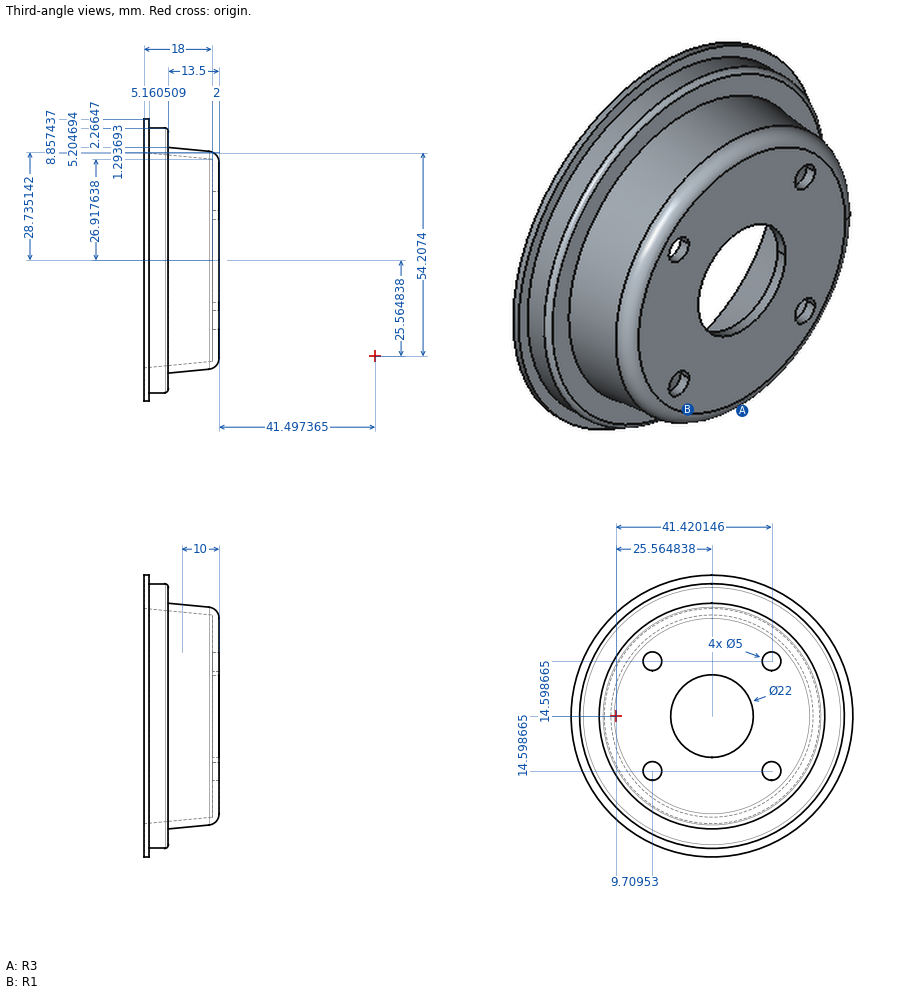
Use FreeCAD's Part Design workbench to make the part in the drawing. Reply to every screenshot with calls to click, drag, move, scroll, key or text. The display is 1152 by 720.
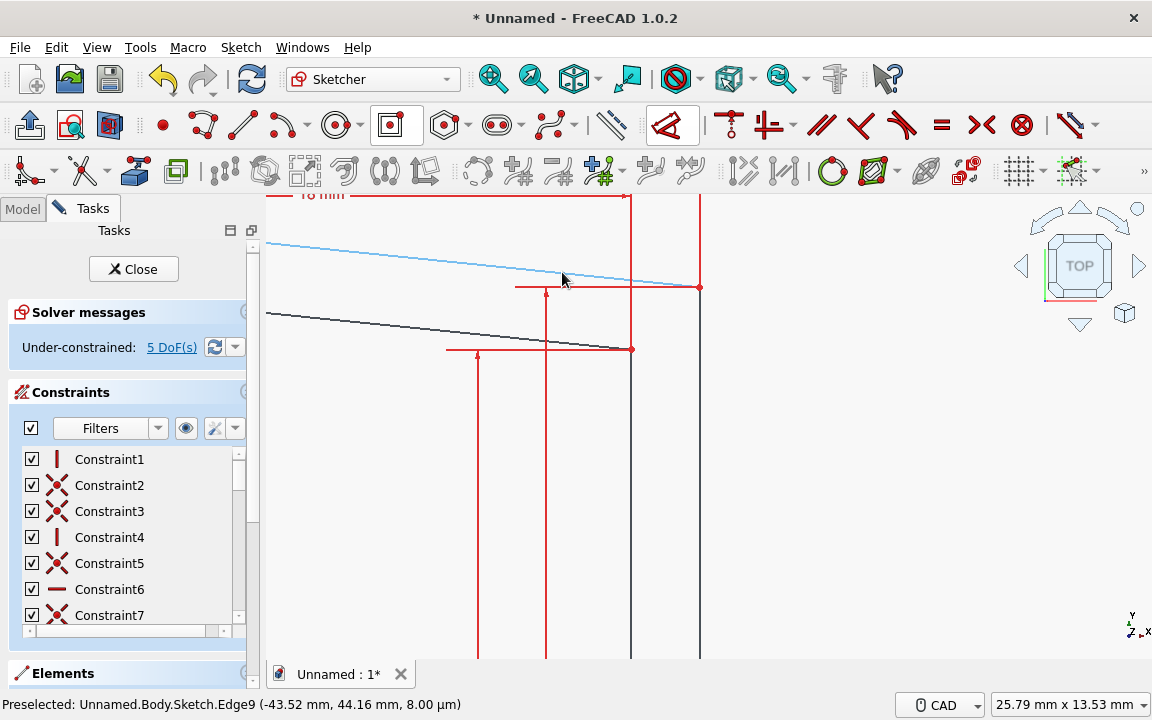
click(561, 273)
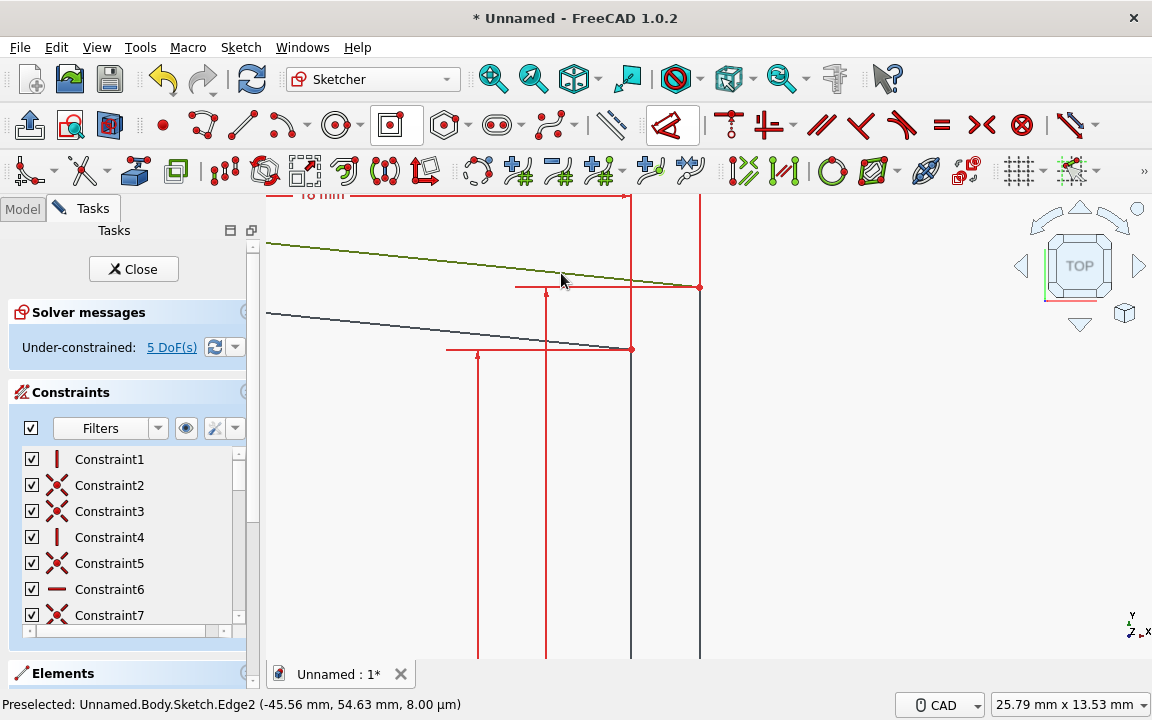
key(i)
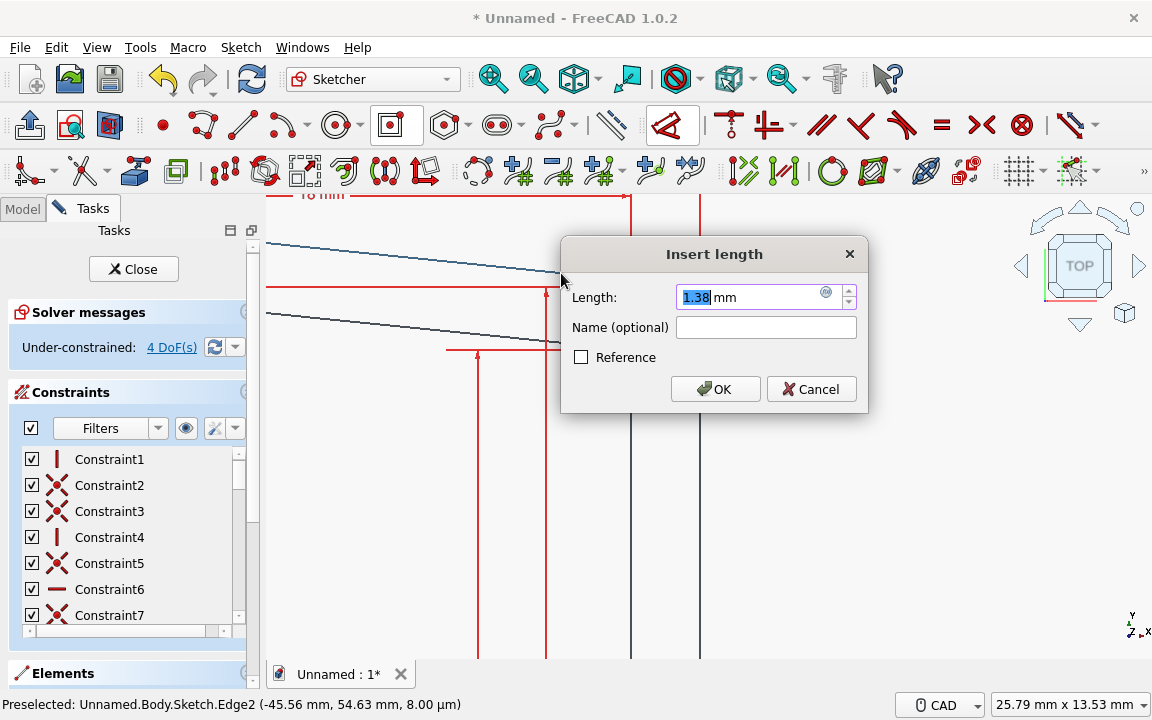
text(1.293693)
key(Return)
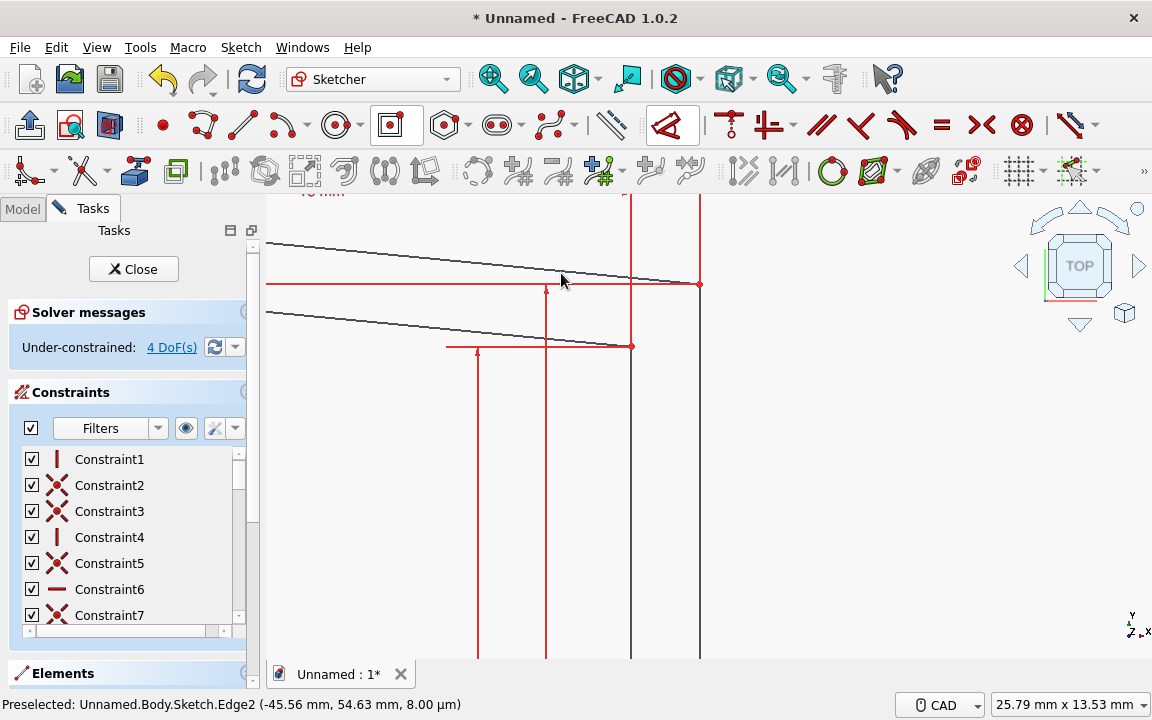
scroll(573, 326, down, 10)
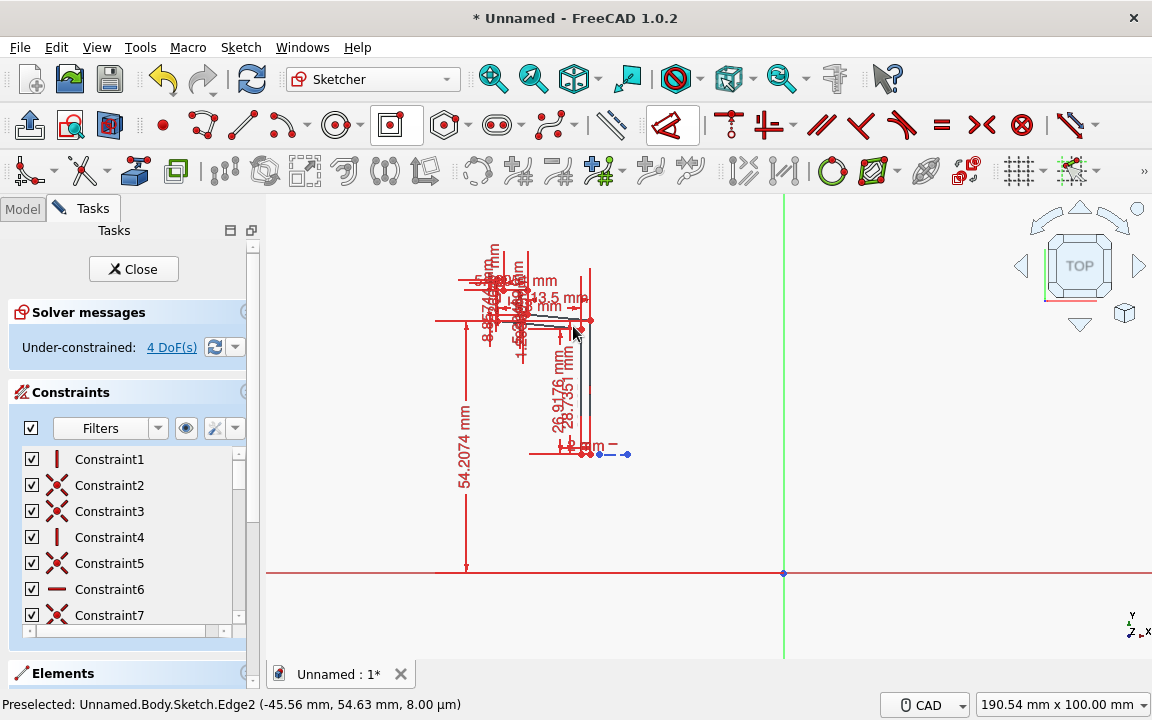
scroll(590, 454, up, 2)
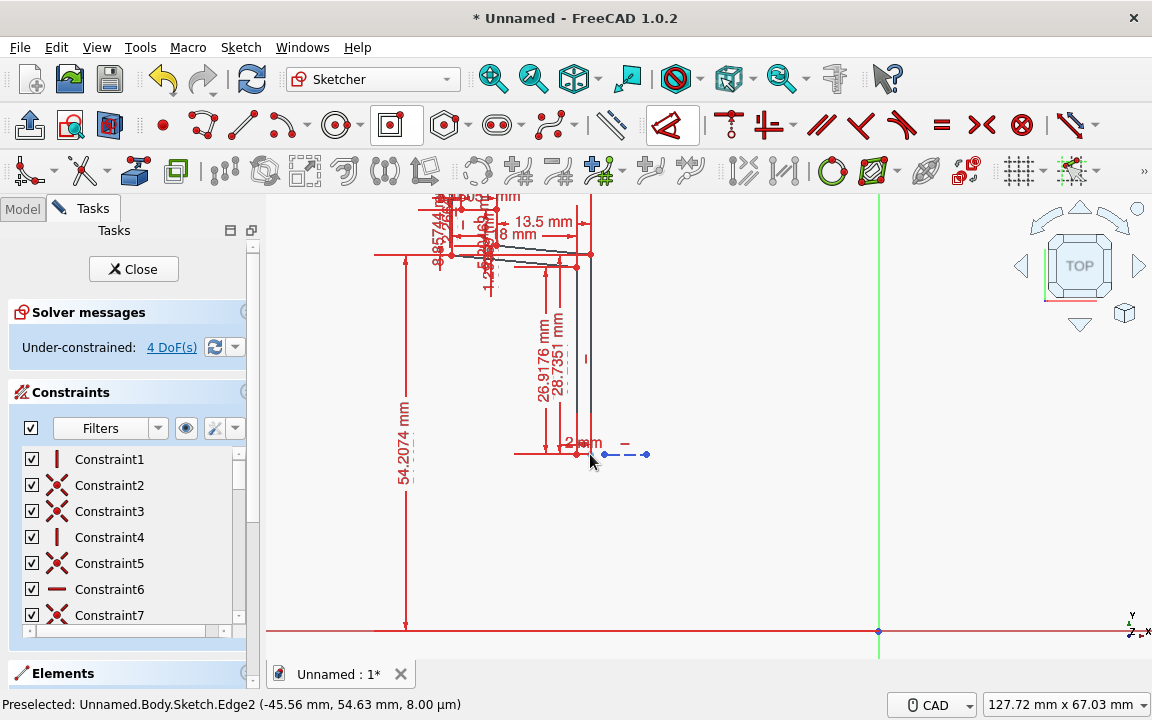
click(591, 454)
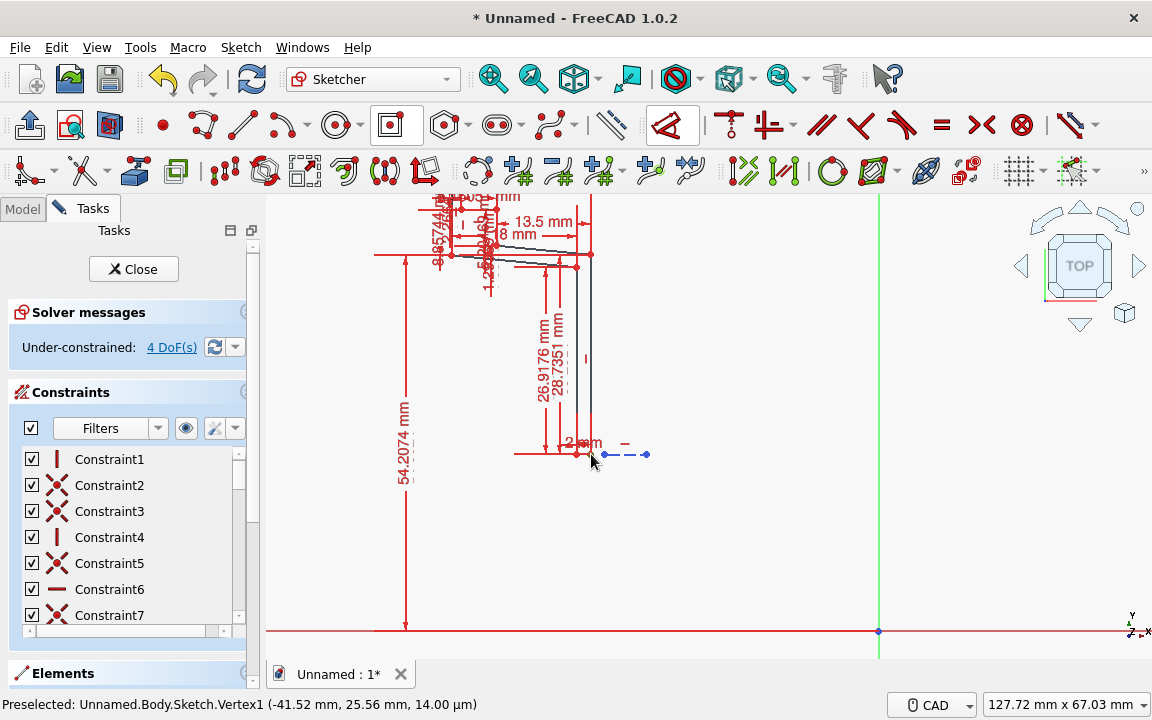
key(l)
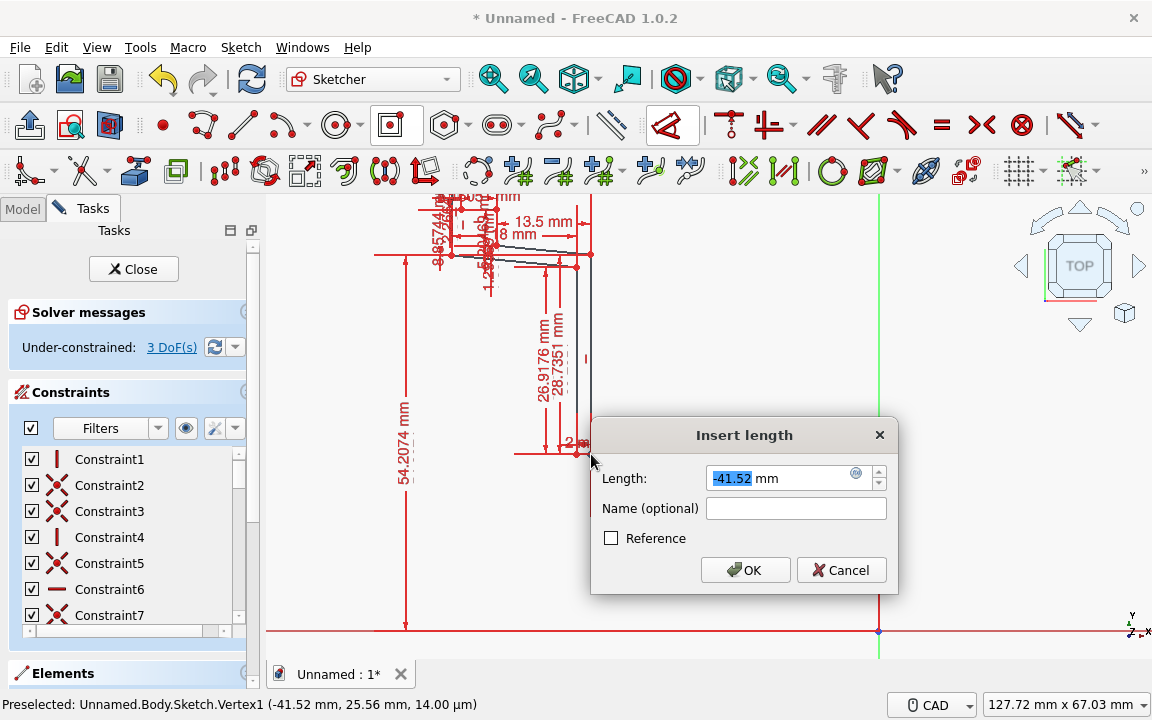
text(-41.497365)
key(Return)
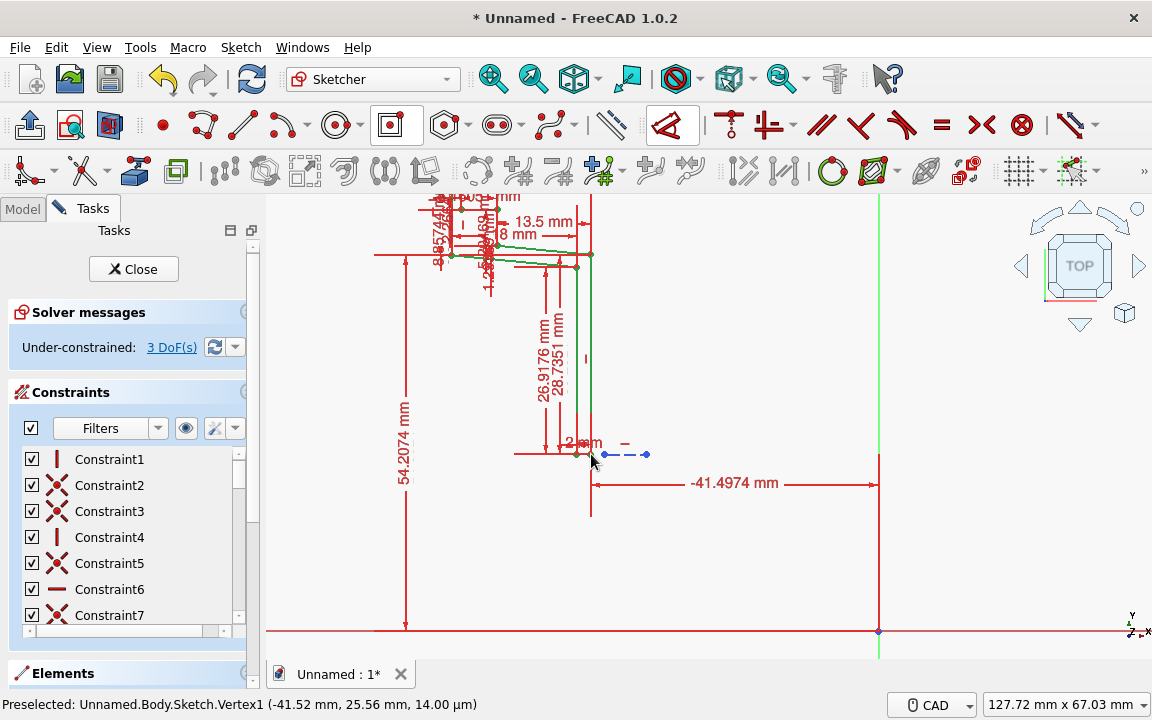
click(604, 455)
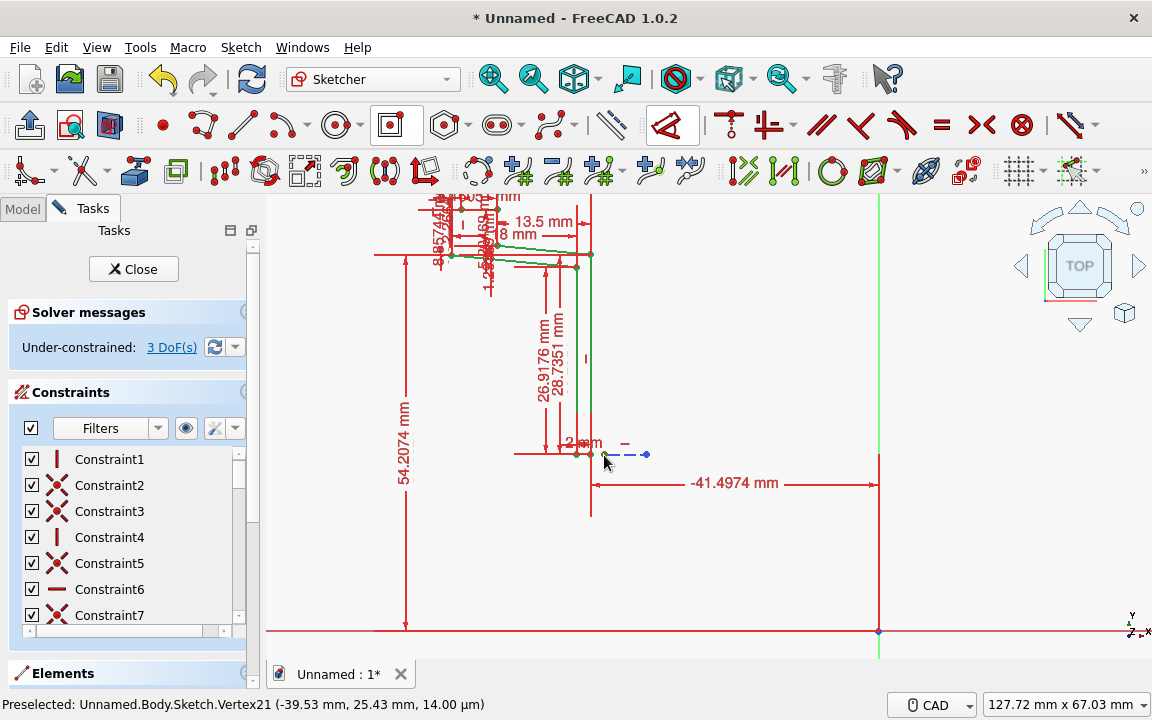
key(i)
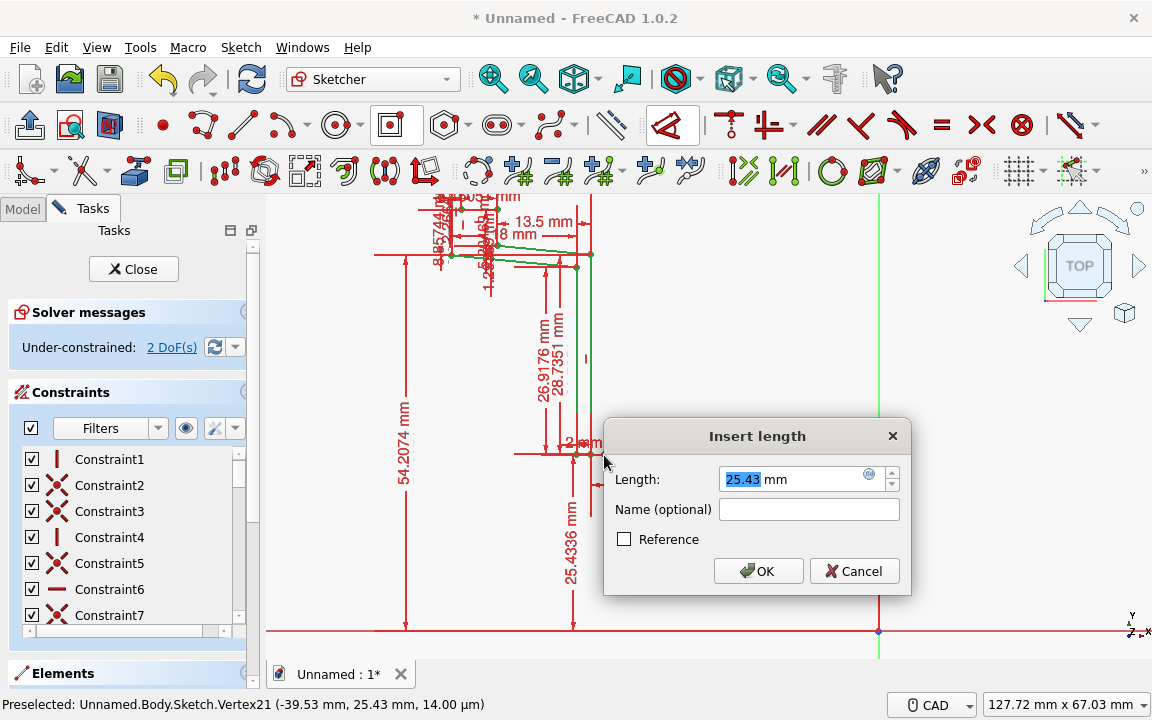
text(25.564838)
key(Return)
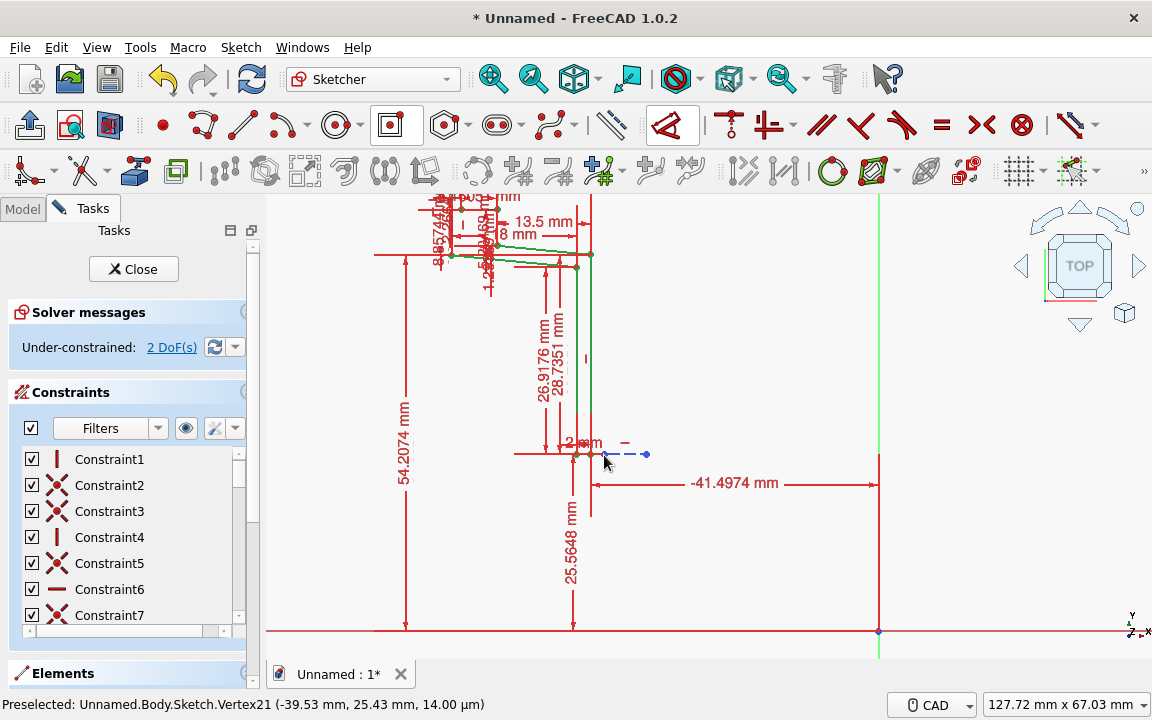
click(134, 269)